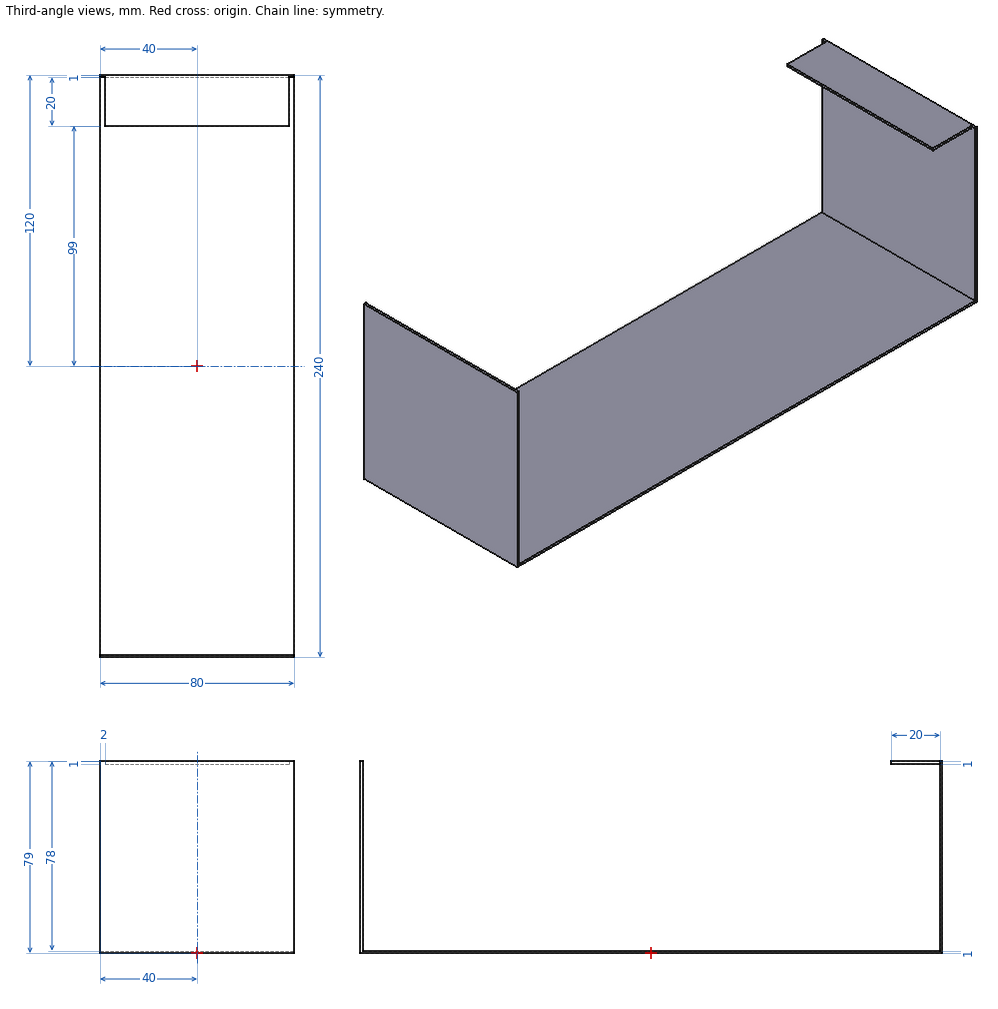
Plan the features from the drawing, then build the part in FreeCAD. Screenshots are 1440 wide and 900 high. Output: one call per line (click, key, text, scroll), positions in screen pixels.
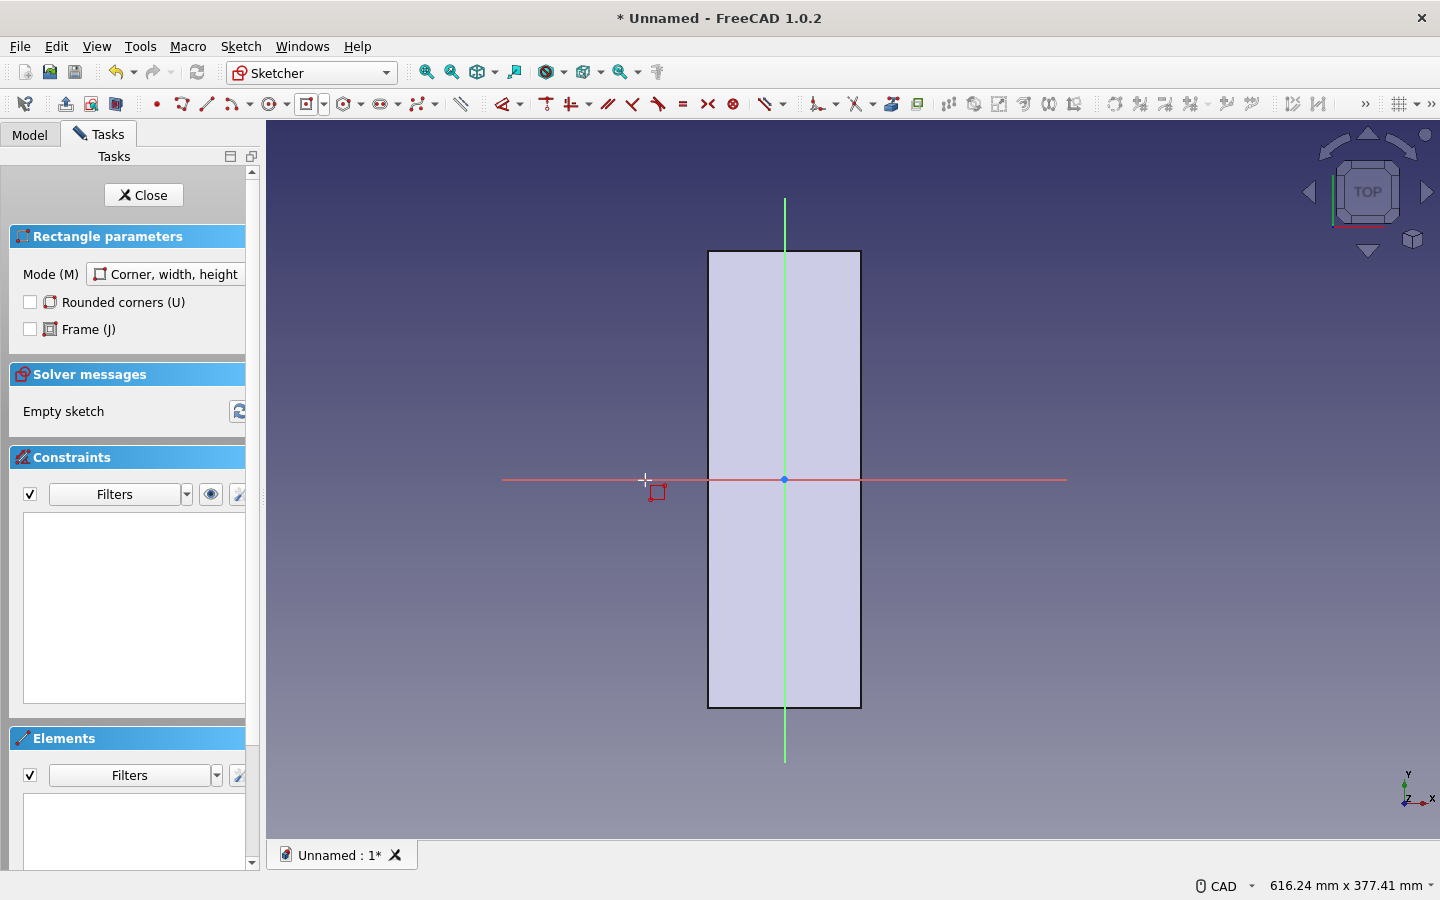
scroll(708, 251, up, 11)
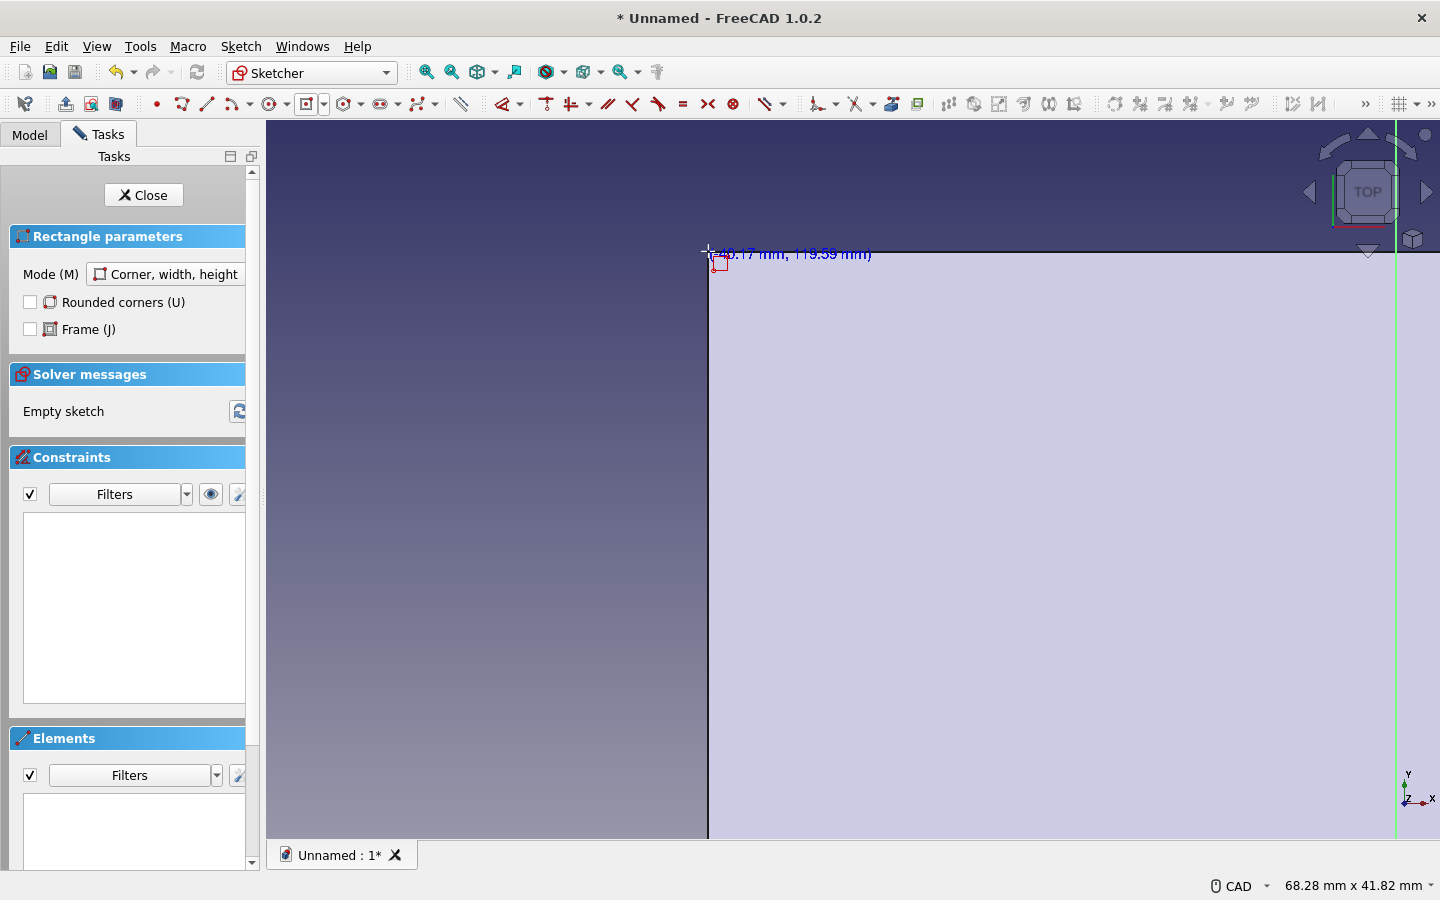
scroll(708, 251, down, 11)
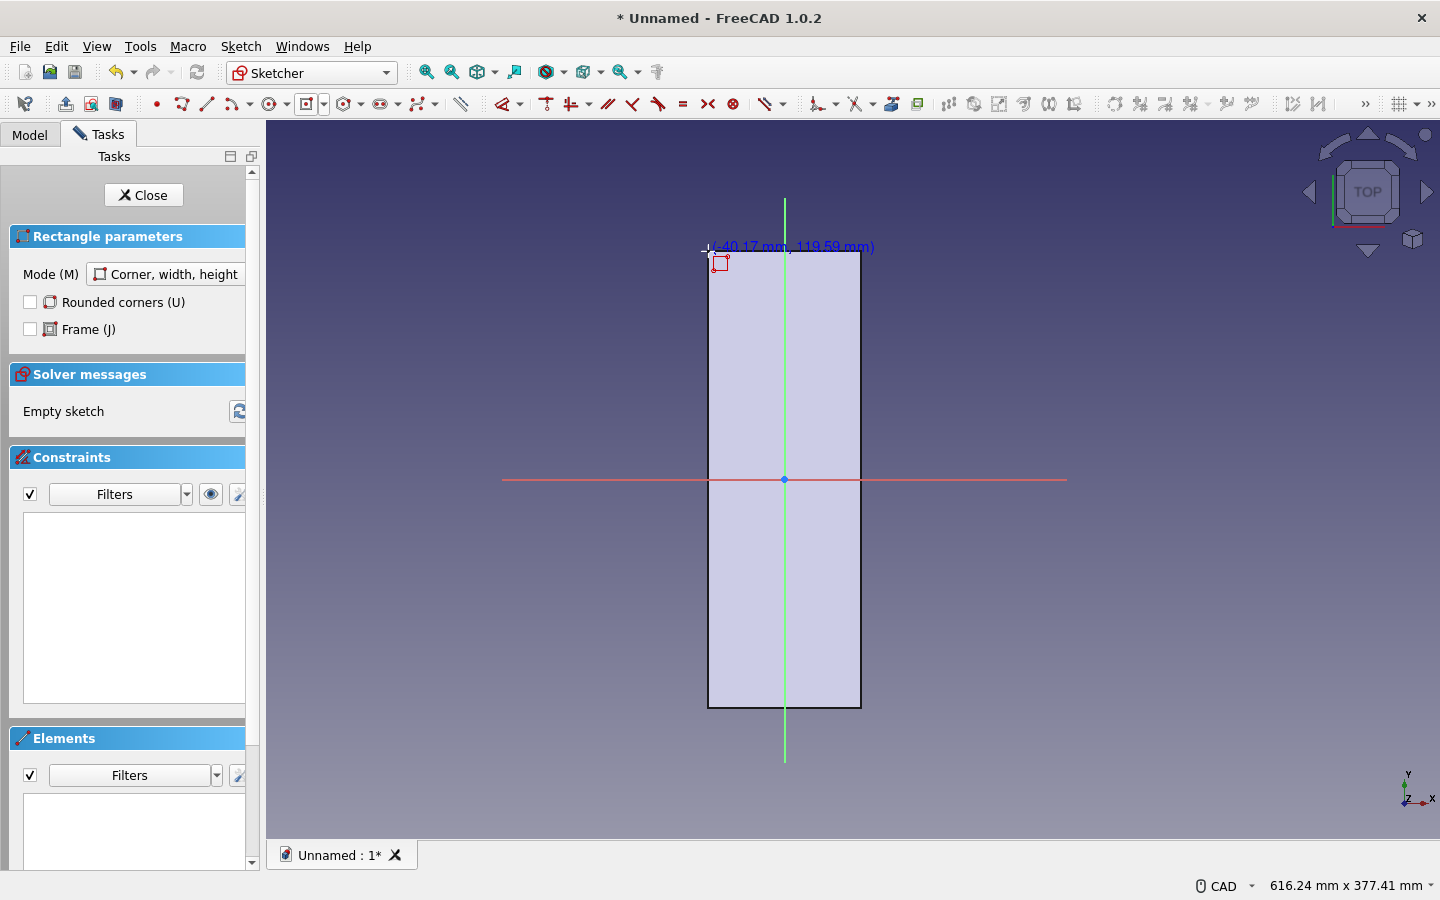
click(708, 251)
click(861, 253)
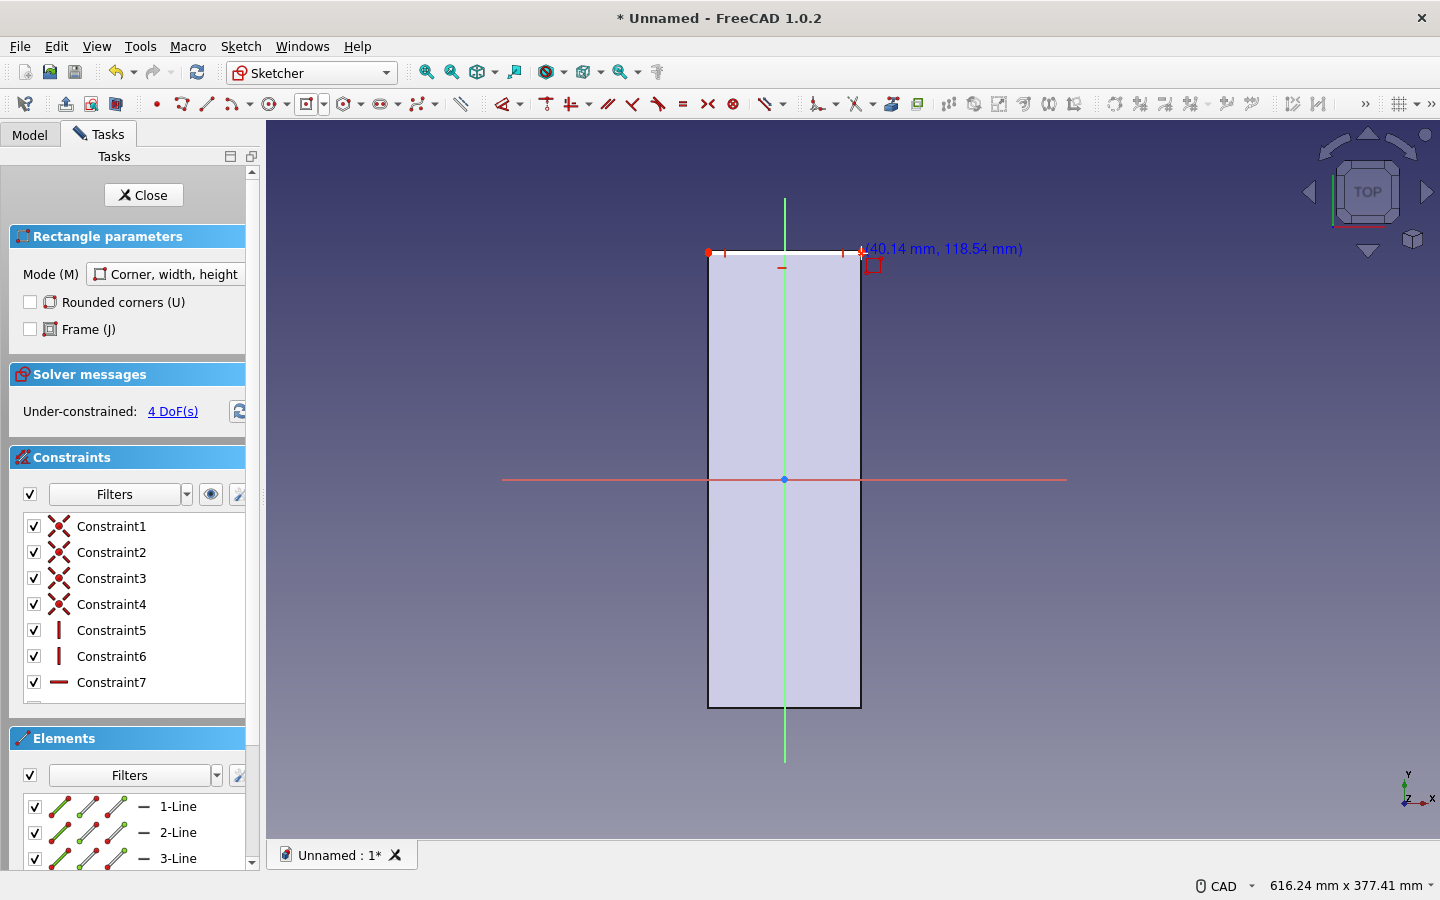
scroll(708, 707, up, 11)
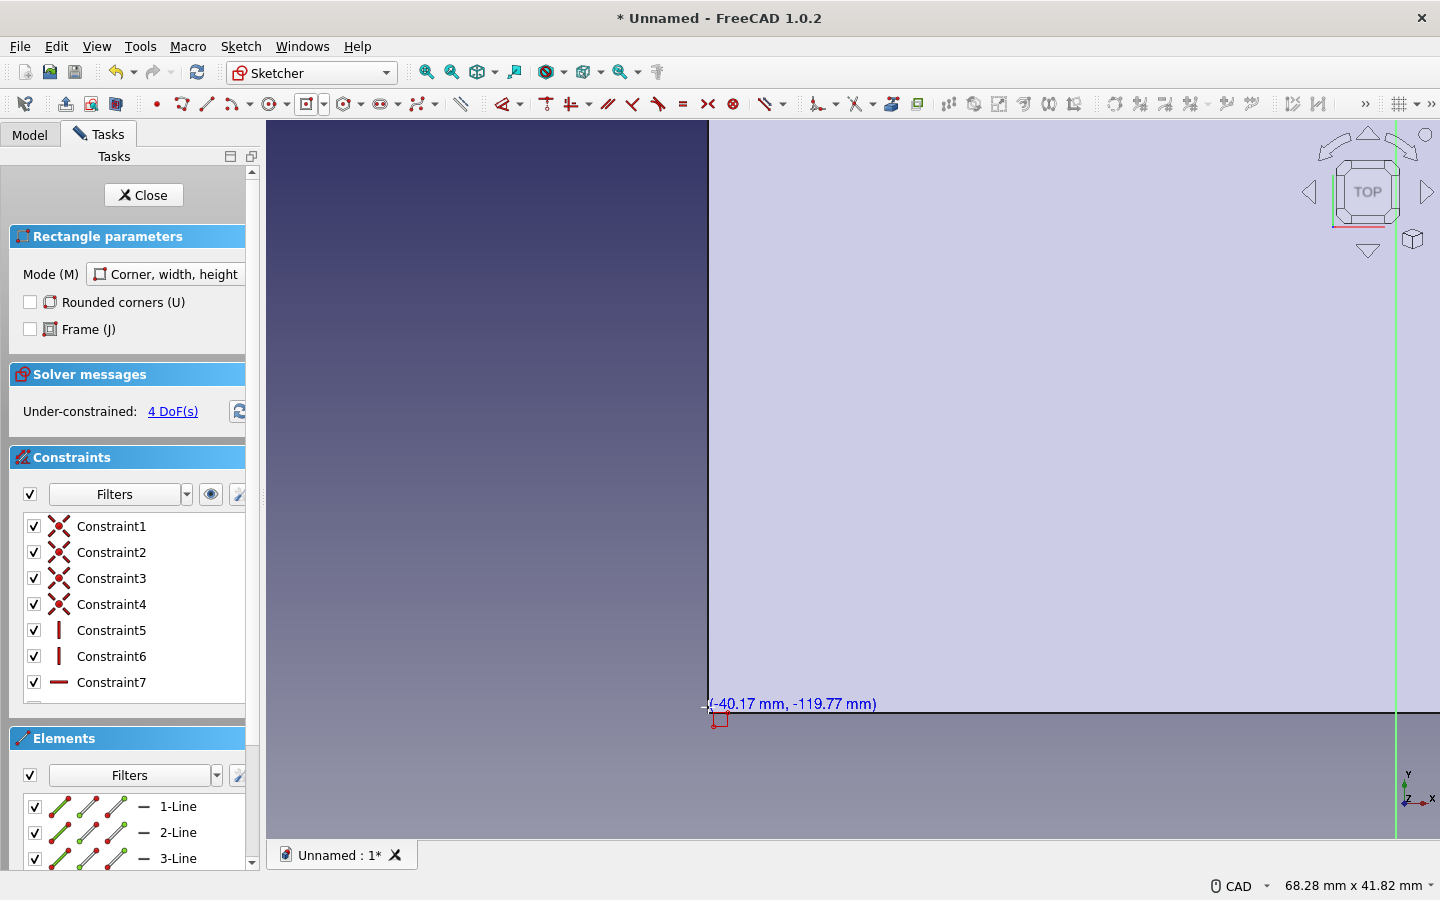
scroll(708, 707, down, 11)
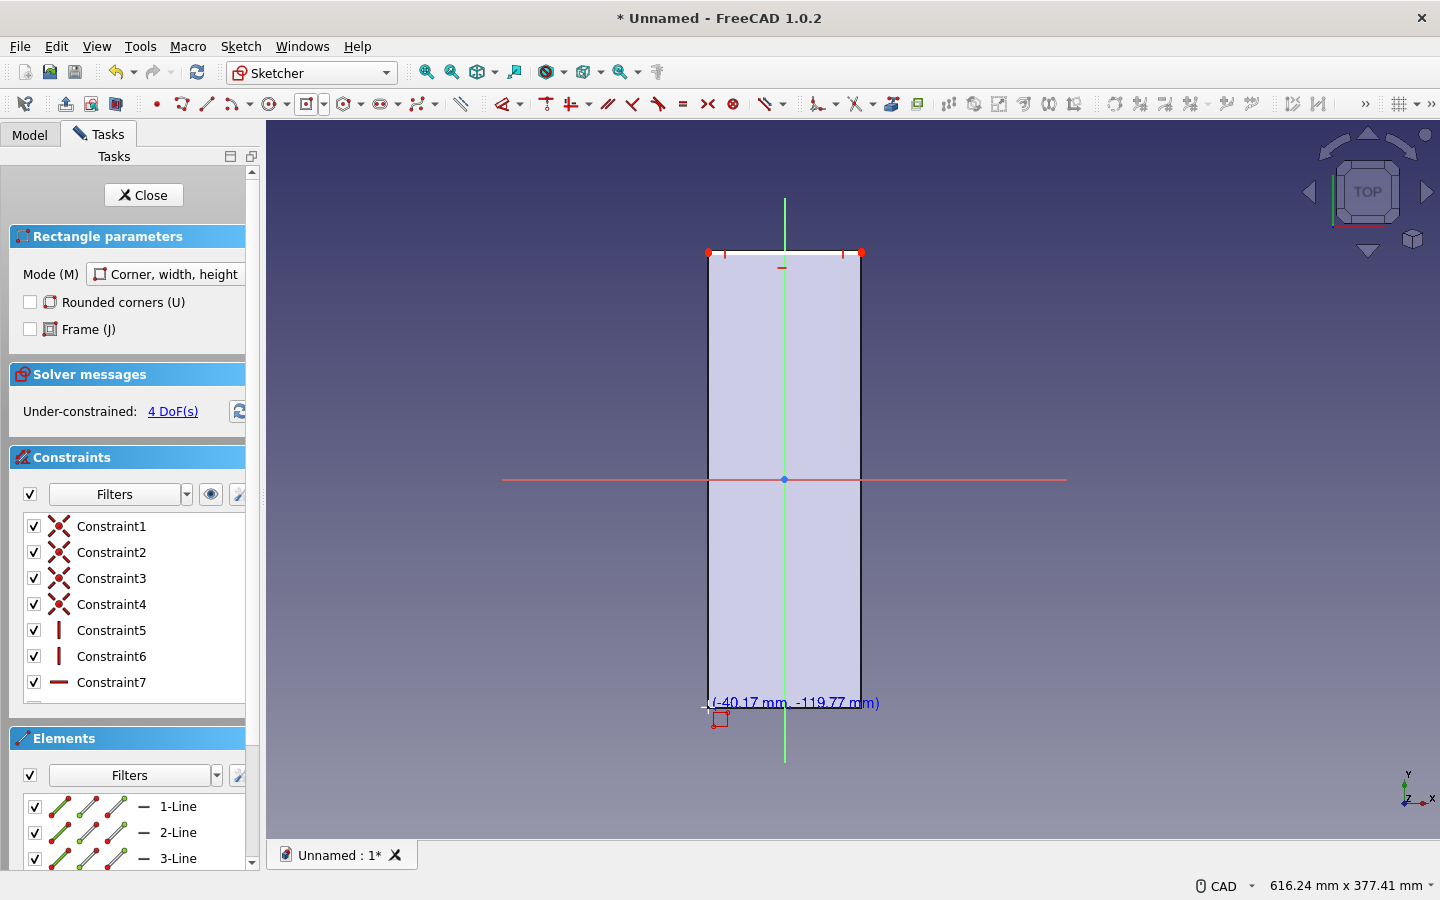
click(708, 707)
click(861, 708)
key(Escape)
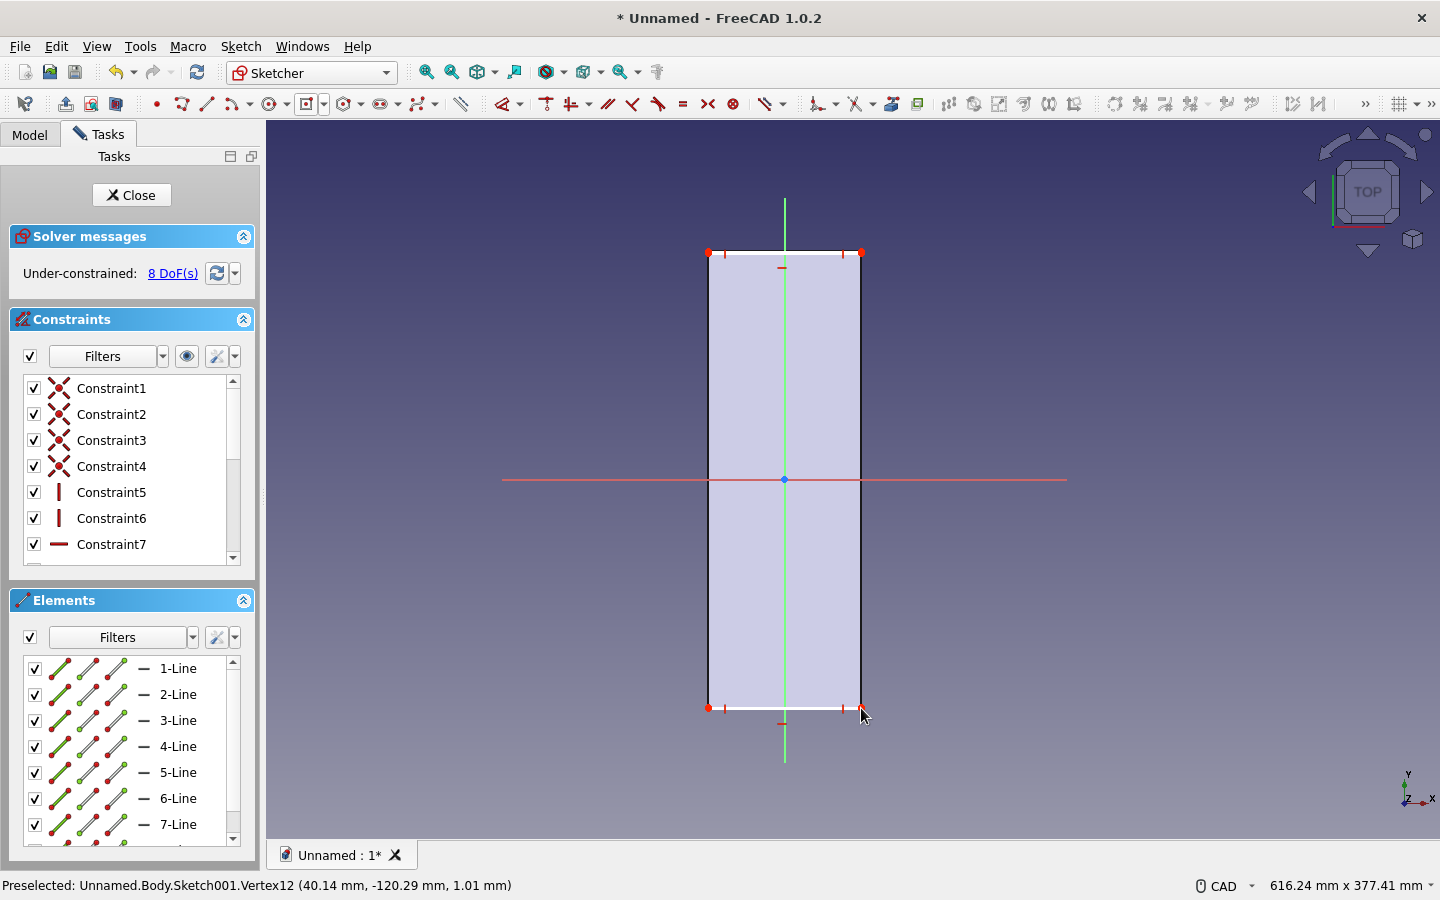
scroll(708, 254, up, 10)